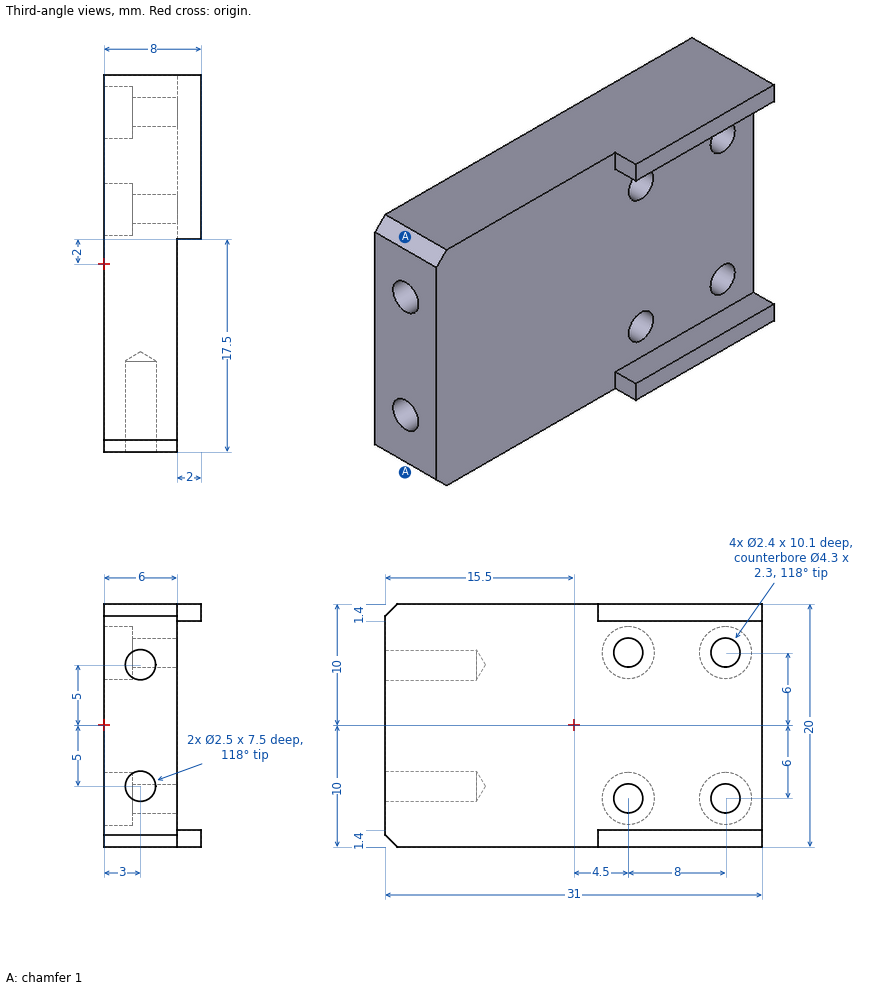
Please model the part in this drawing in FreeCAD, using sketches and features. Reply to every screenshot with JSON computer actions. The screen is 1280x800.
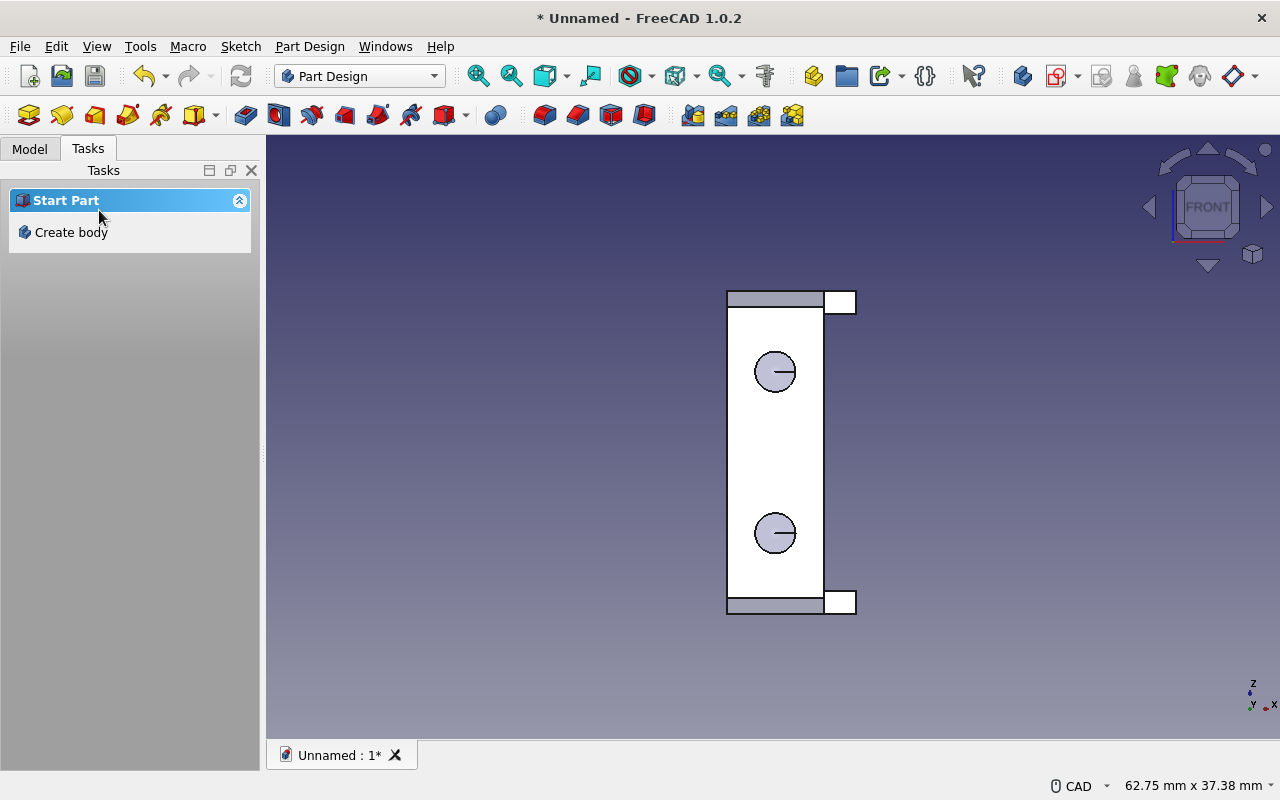
{"action": "key", "text": "0"}